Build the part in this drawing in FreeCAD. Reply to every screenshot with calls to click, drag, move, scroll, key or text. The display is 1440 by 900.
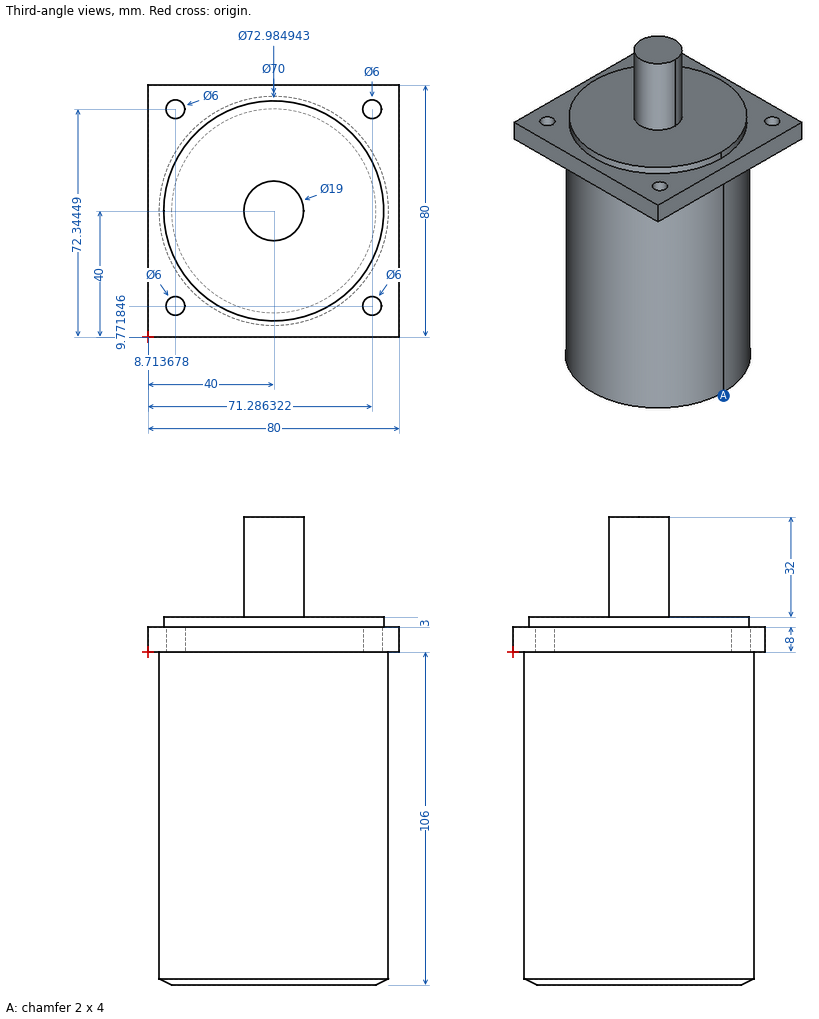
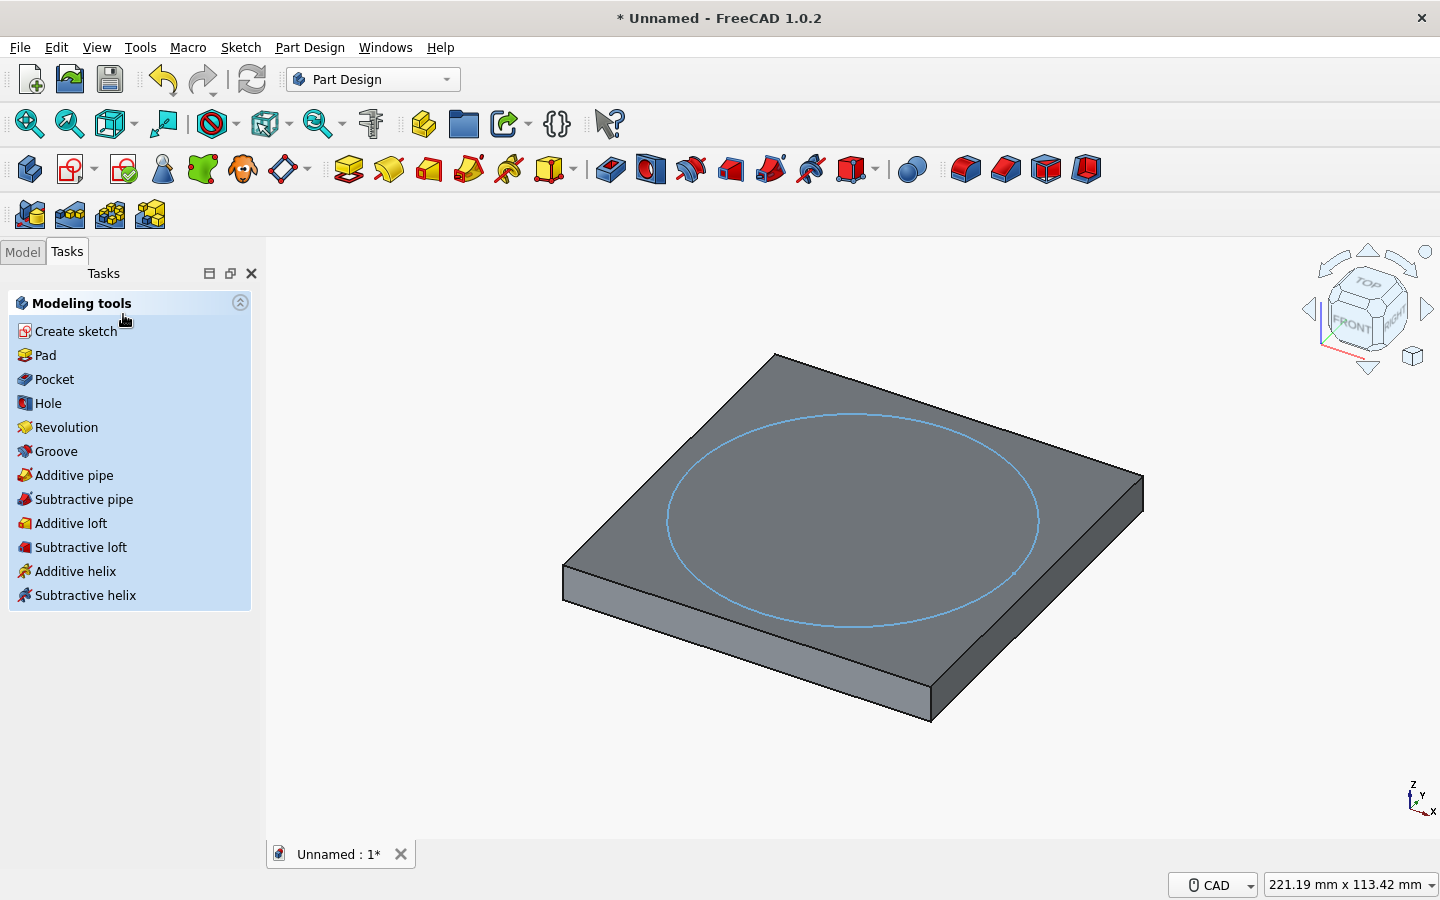
click(350, 170)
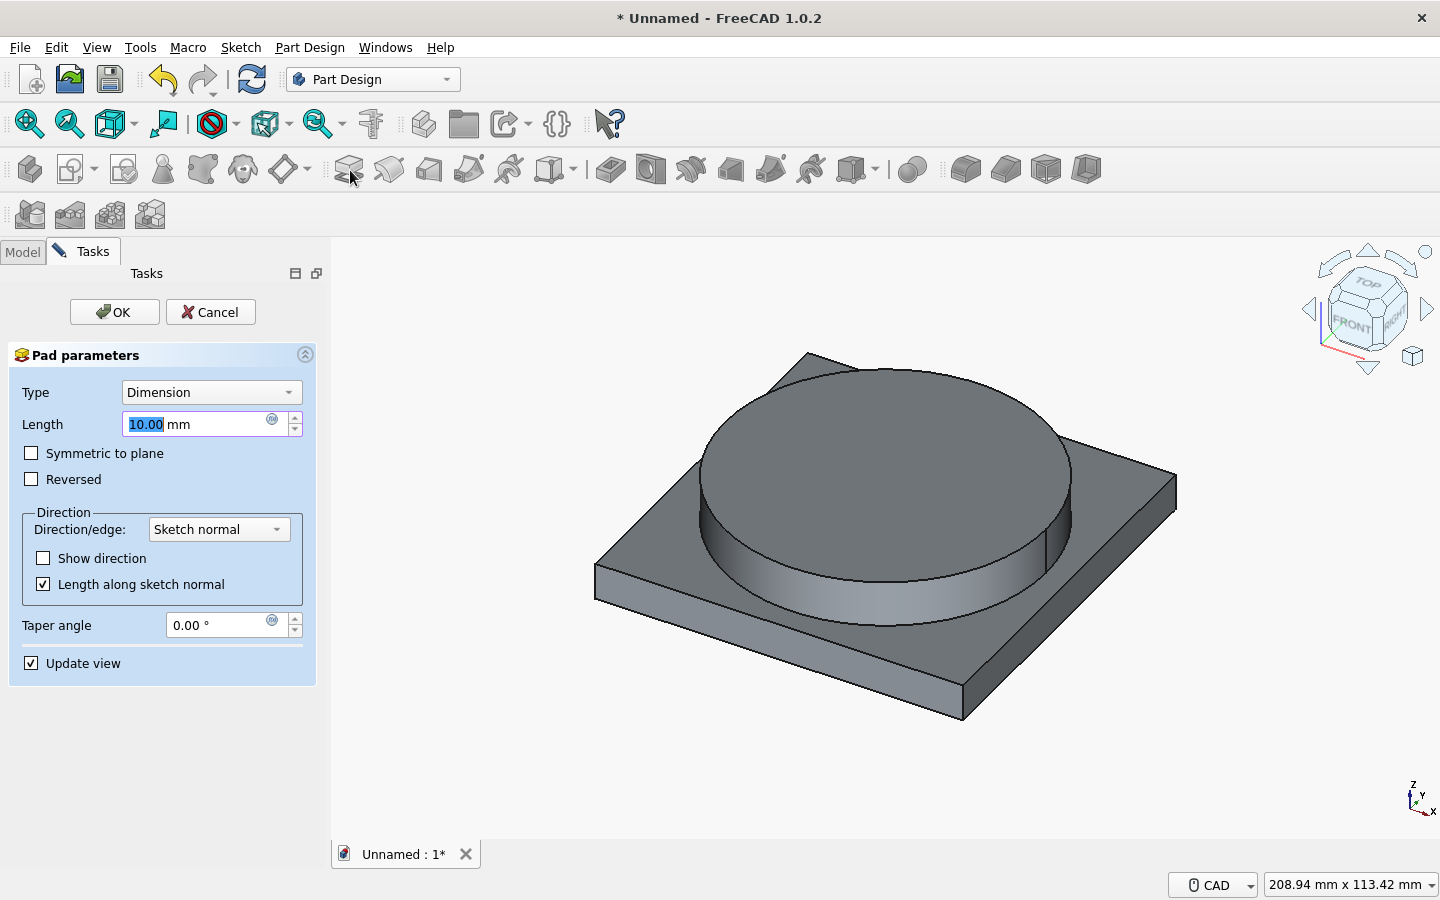
text(3)
key(Tab)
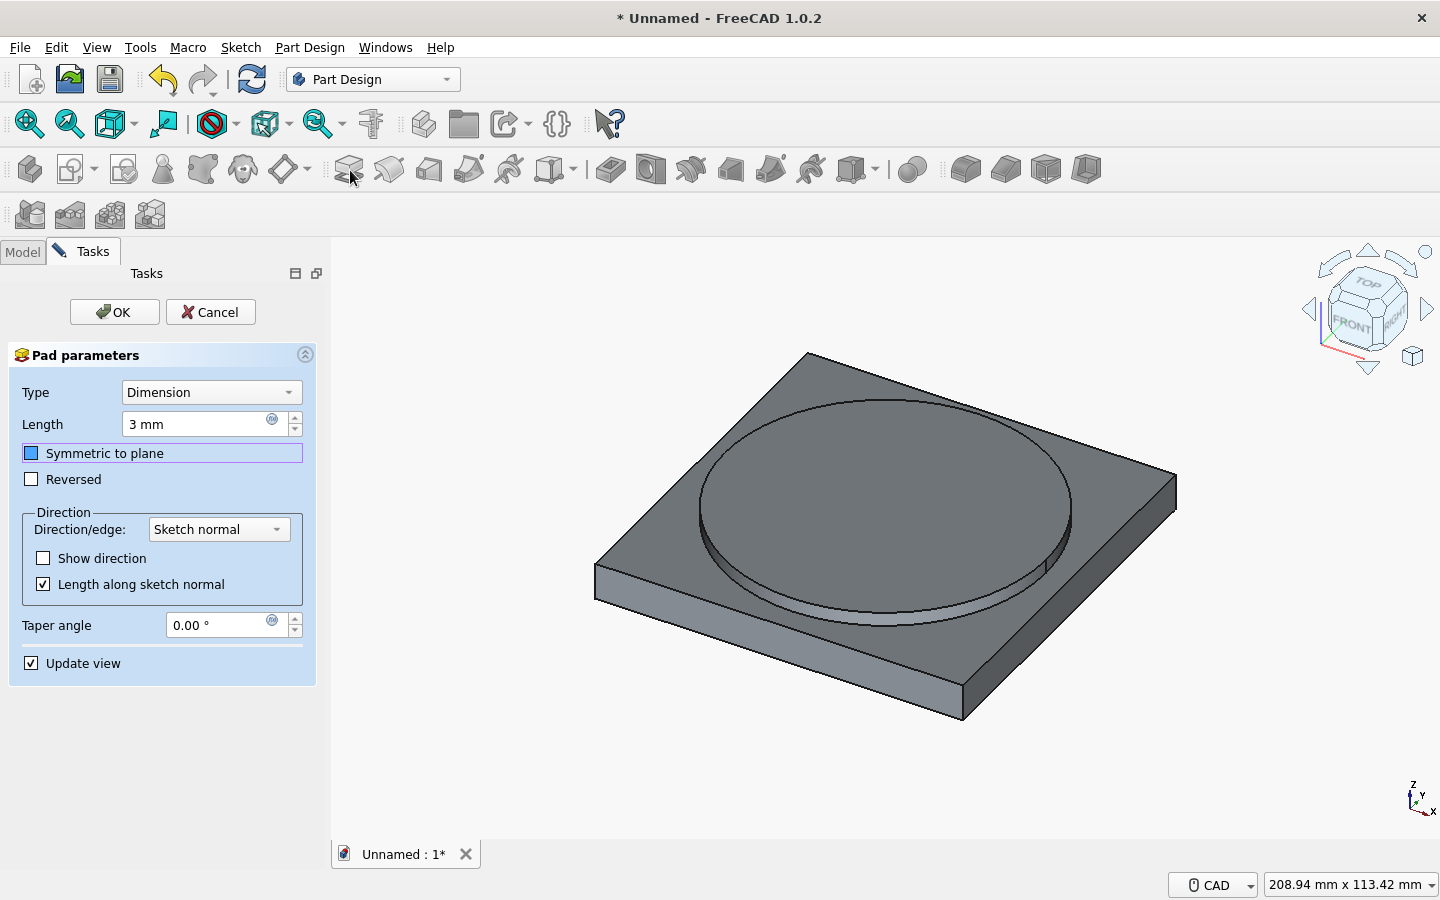
click(115, 312)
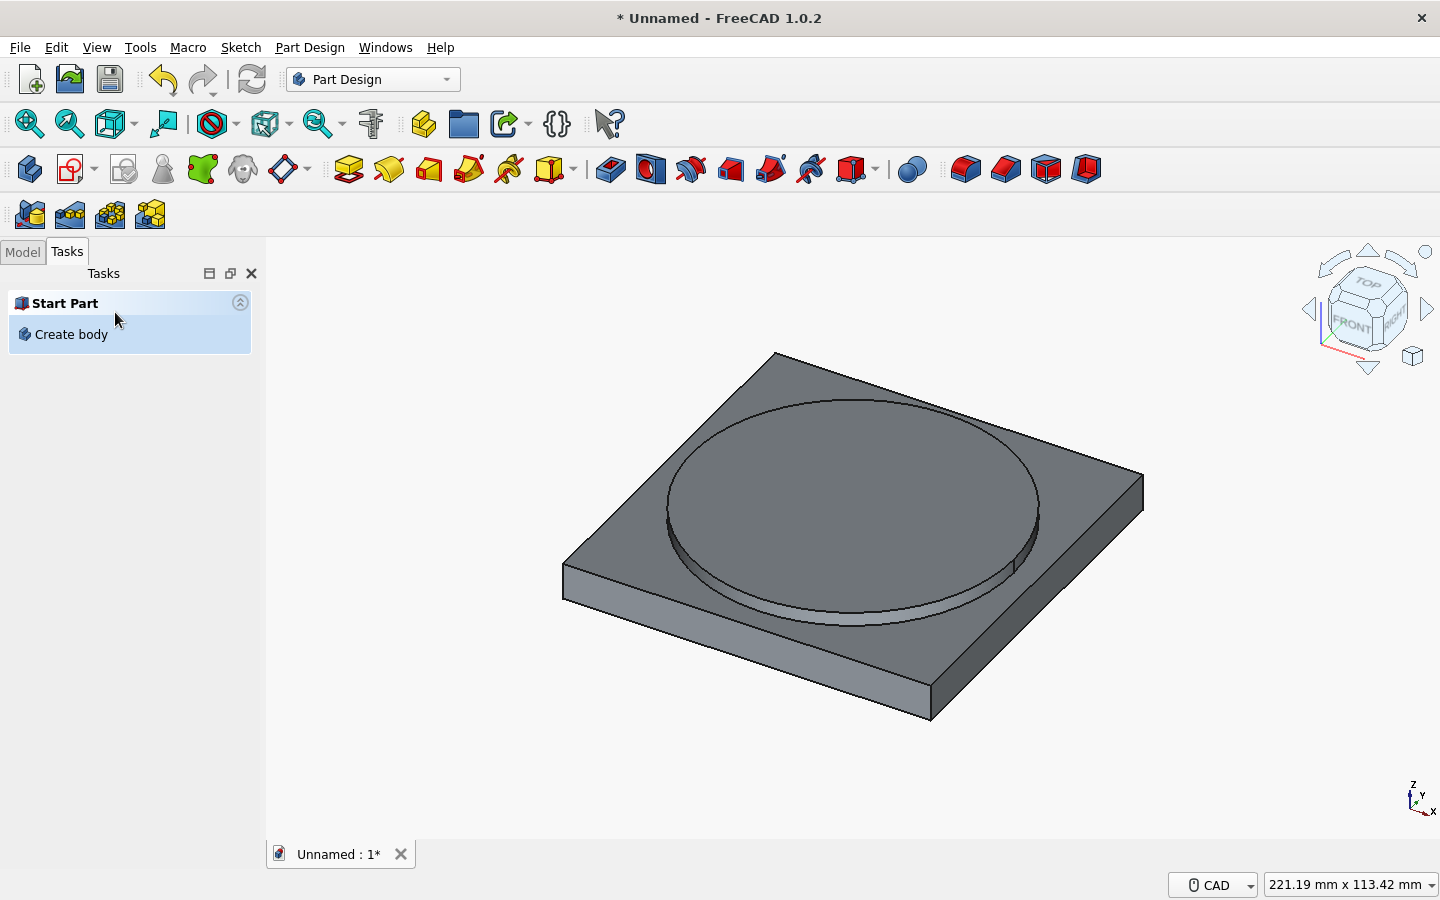
click(853, 505)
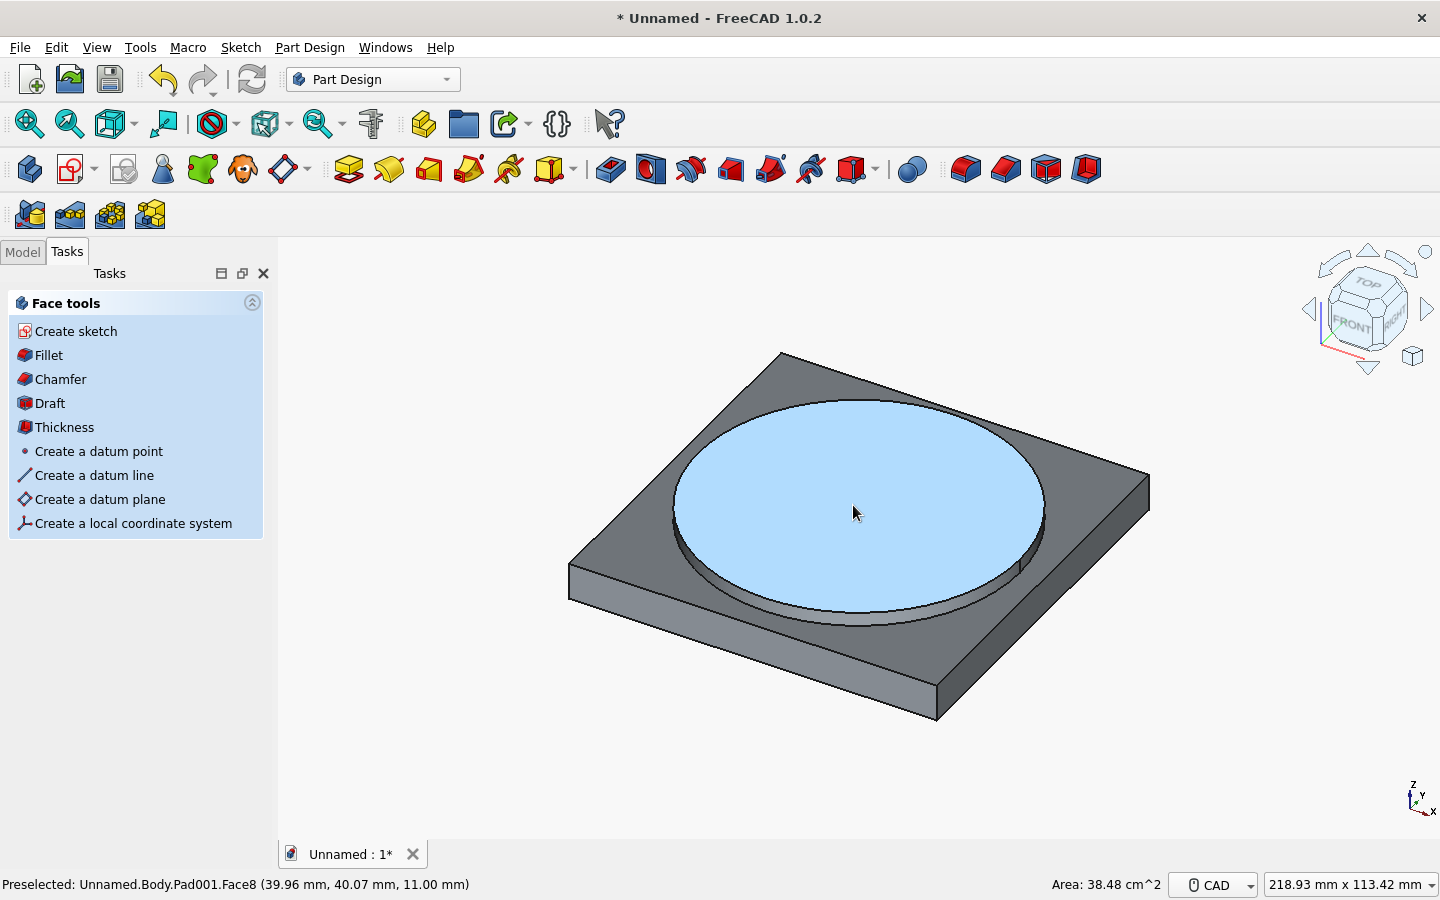
click(70, 170)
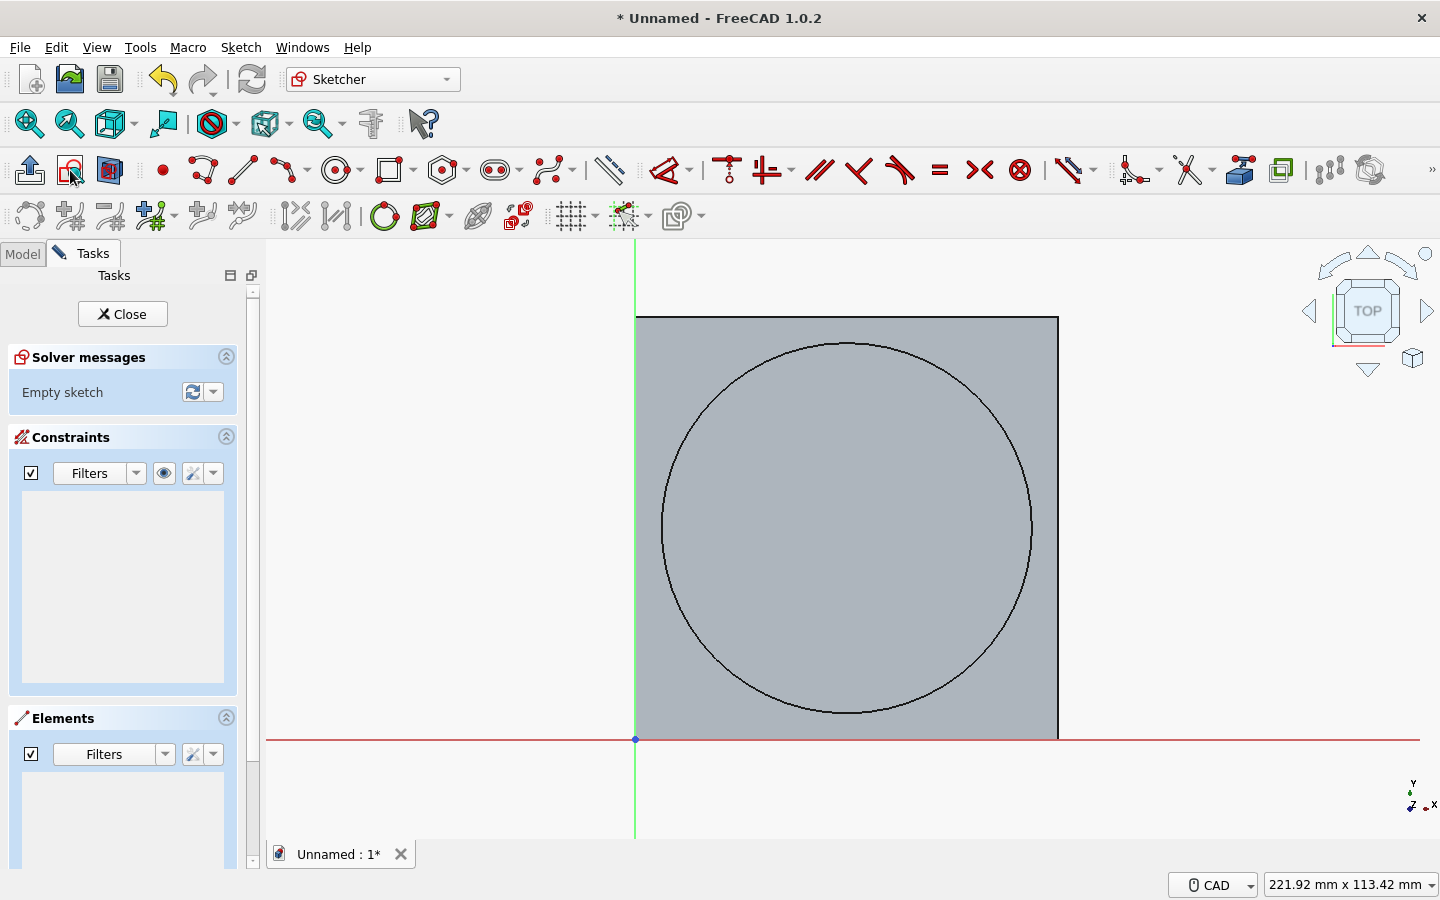
scroll(867, 525, up, 7)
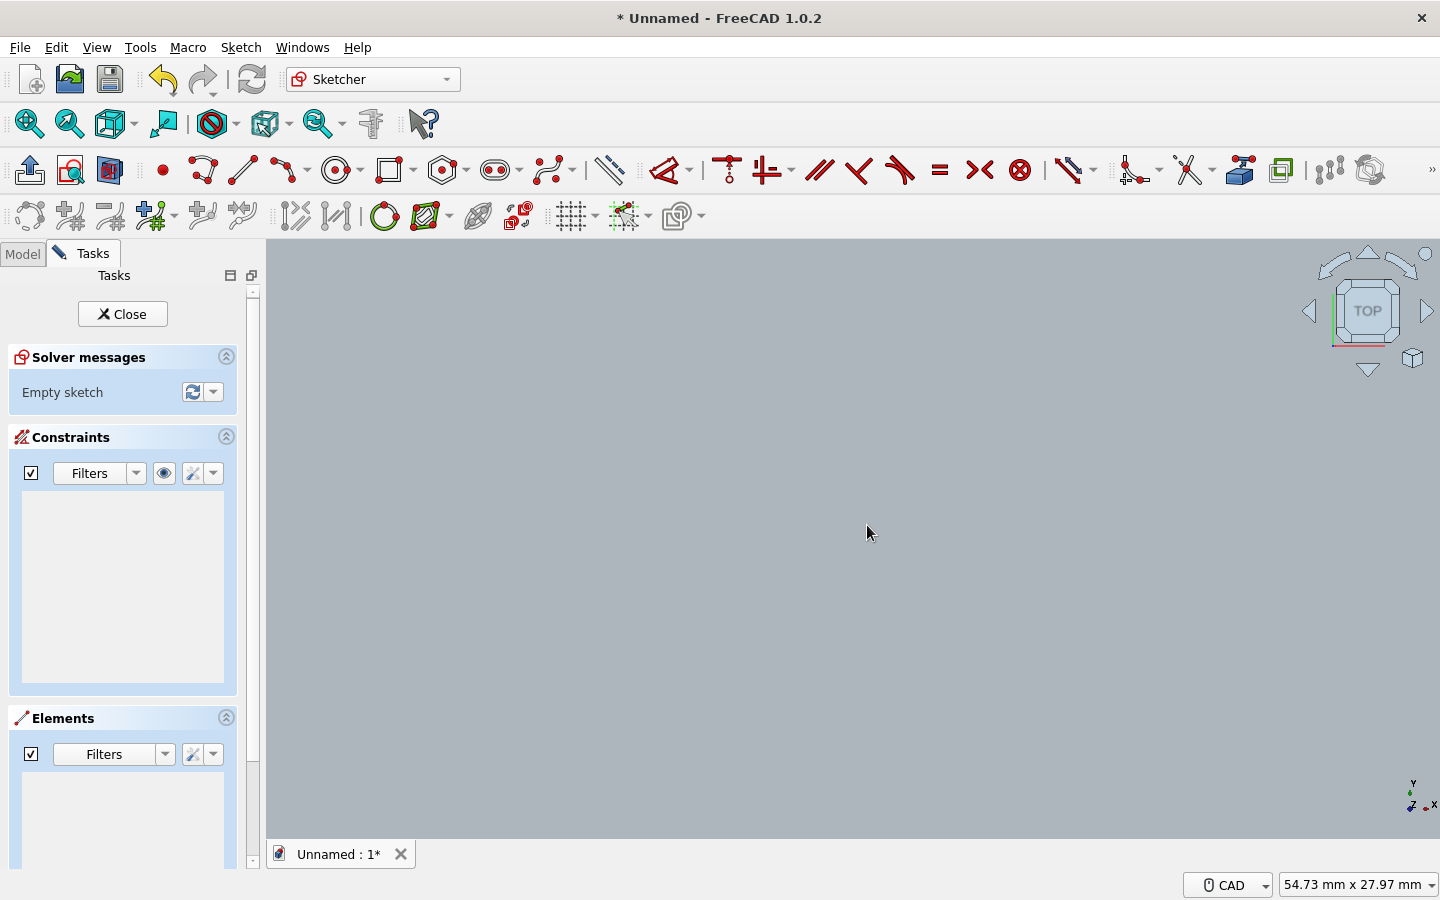
click(336, 170)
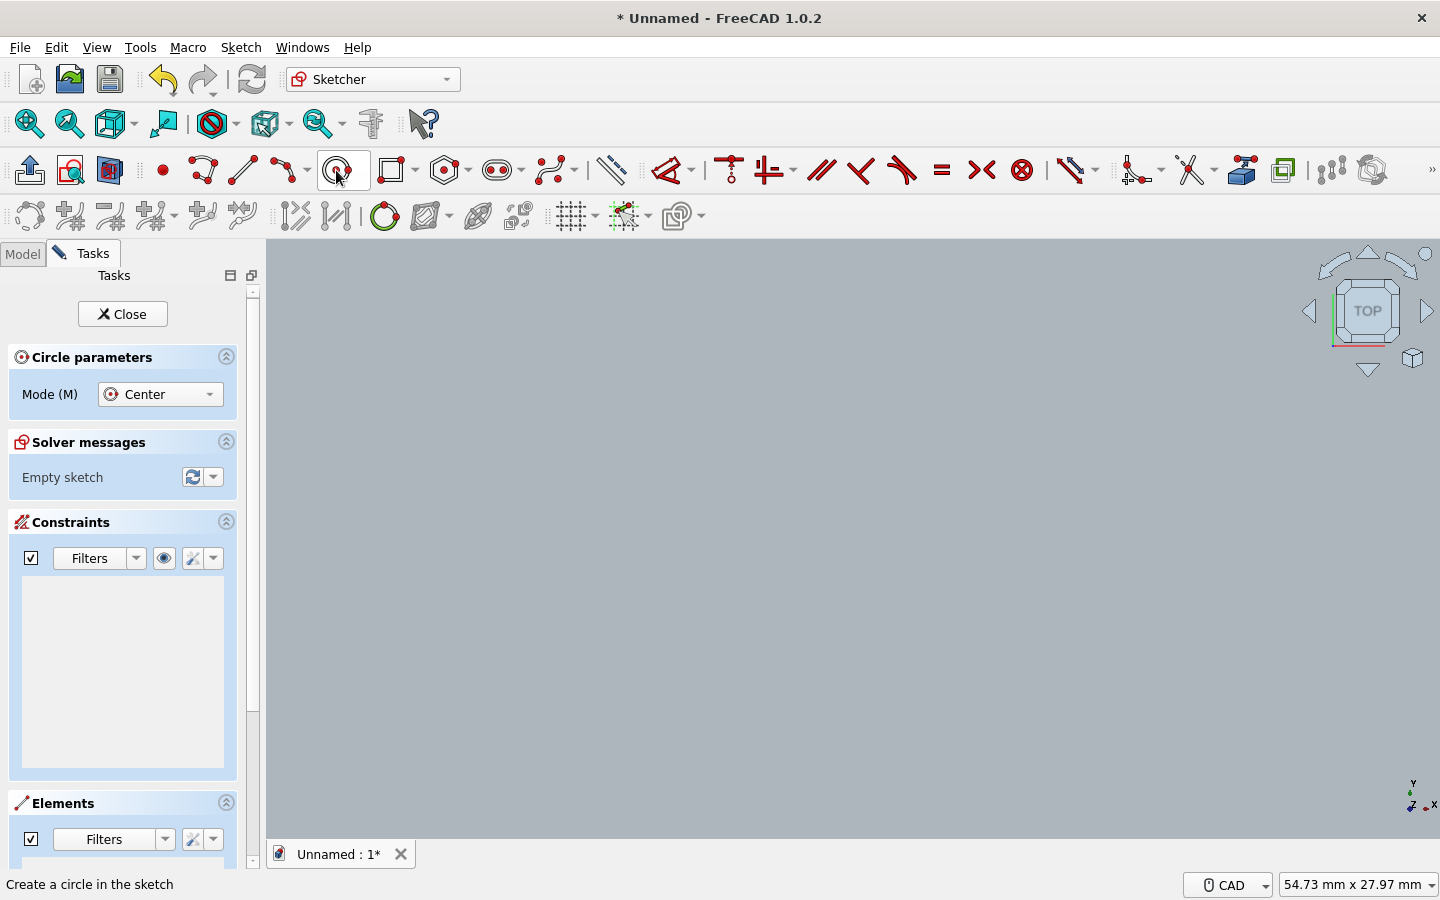
click(783, 537)
move(927, 392)